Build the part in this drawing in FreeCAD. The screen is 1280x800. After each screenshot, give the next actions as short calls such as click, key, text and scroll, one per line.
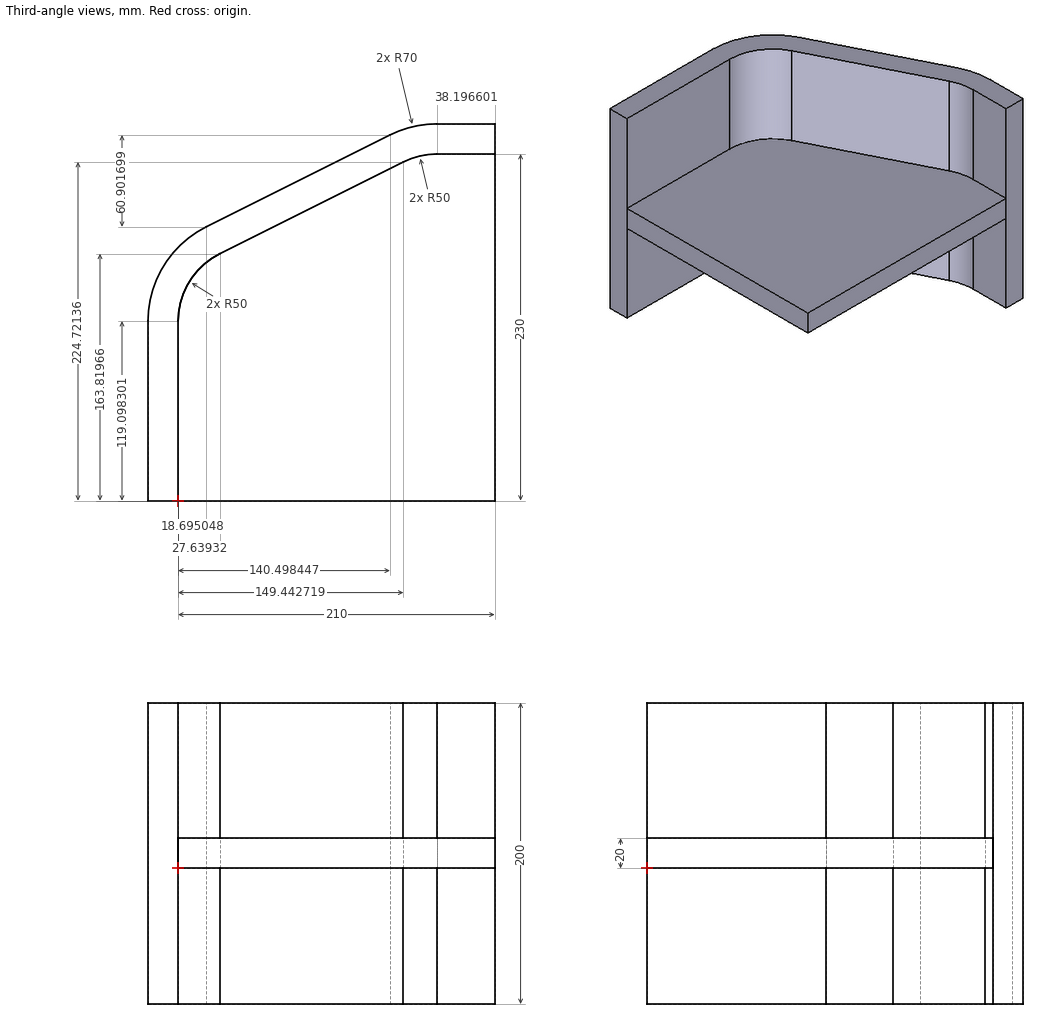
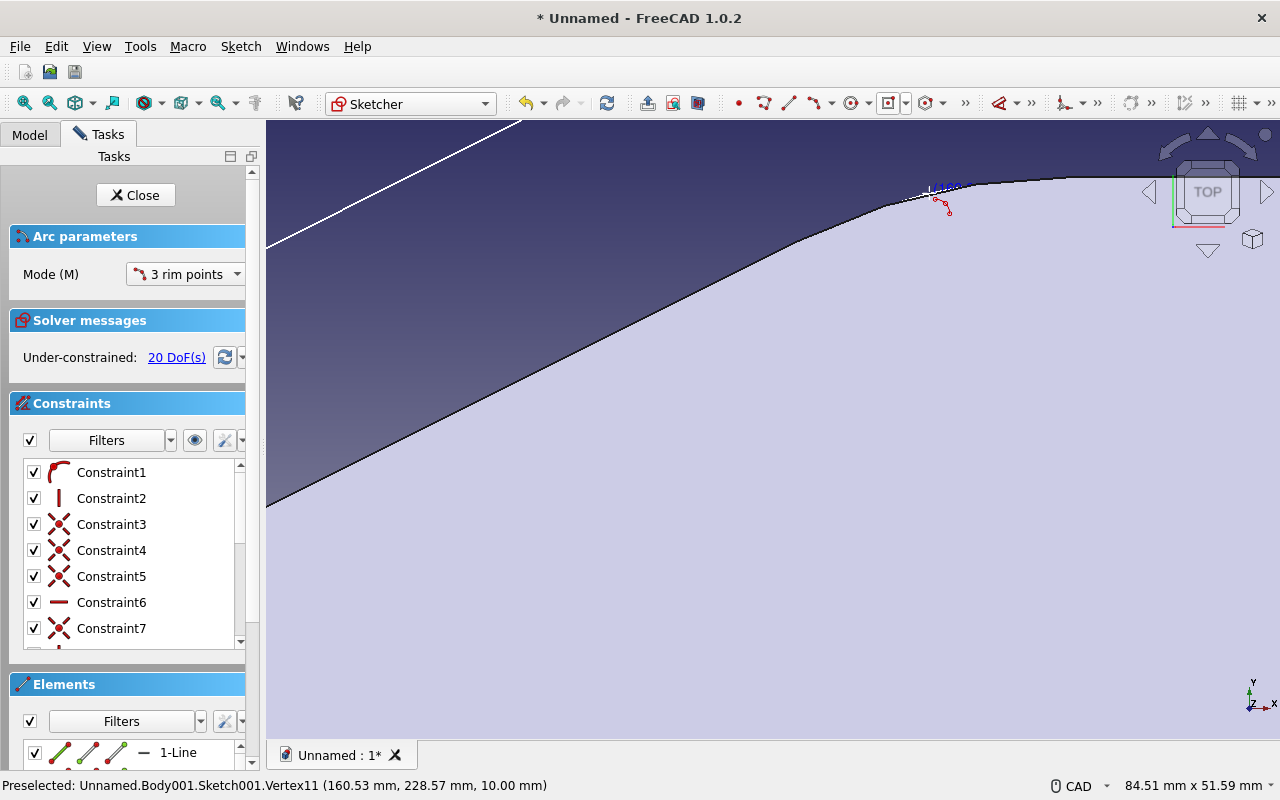
scroll(792, 272, down, 10)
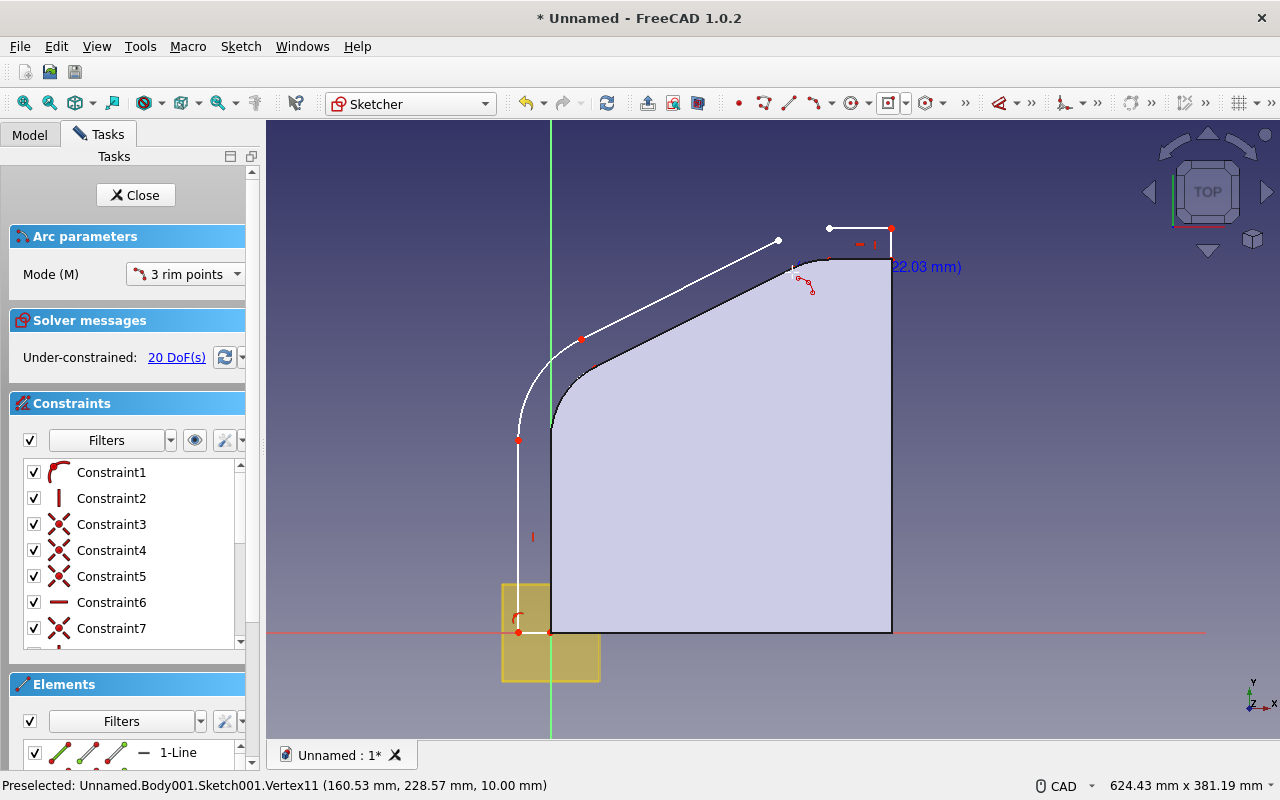
click(829, 228)
click(778, 240)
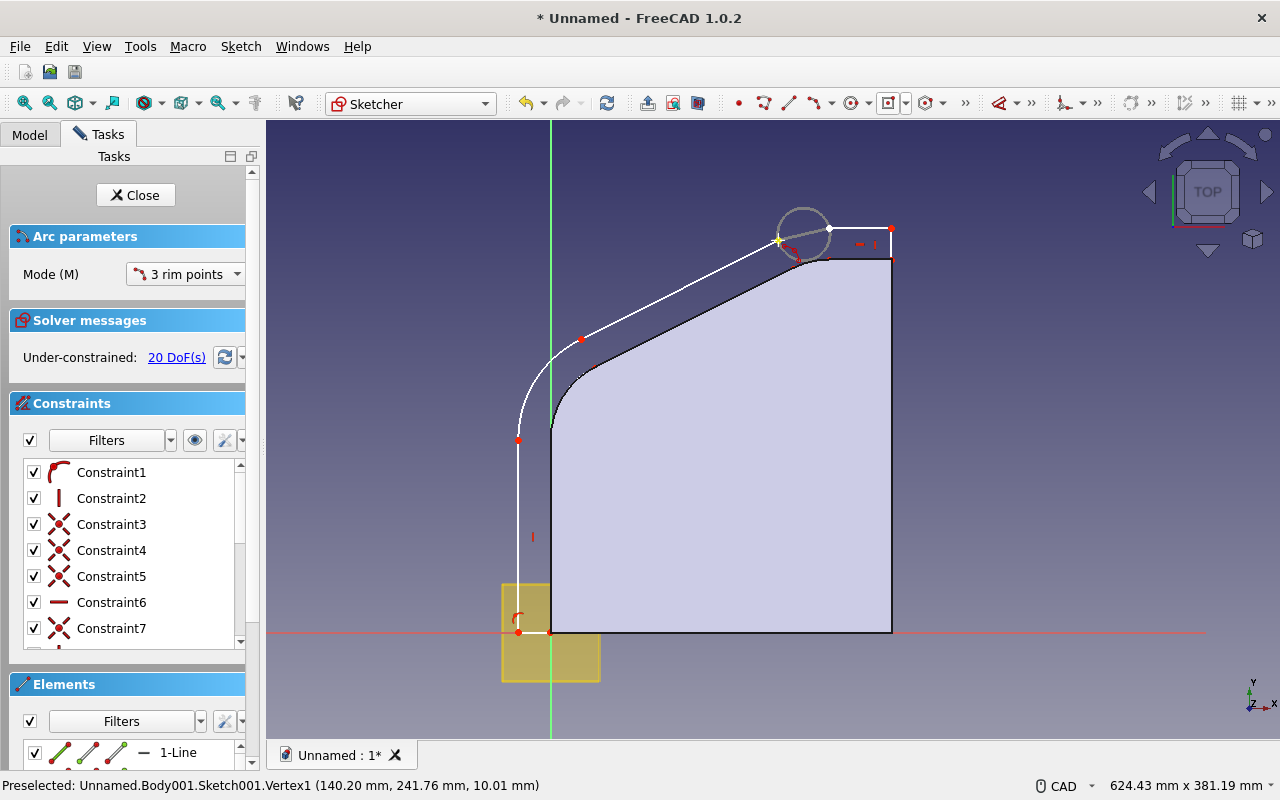
scroll(804, 230, up, 9)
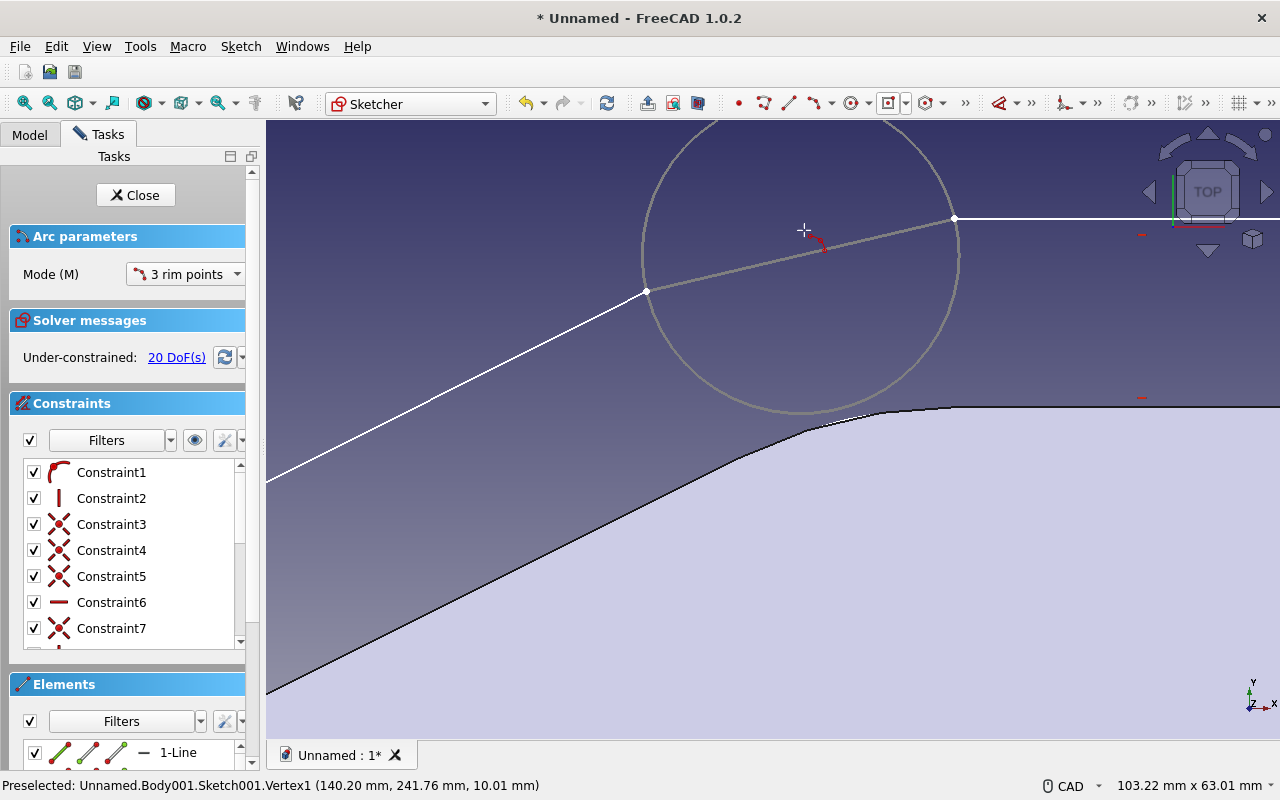
click(799, 229)
key(Escape)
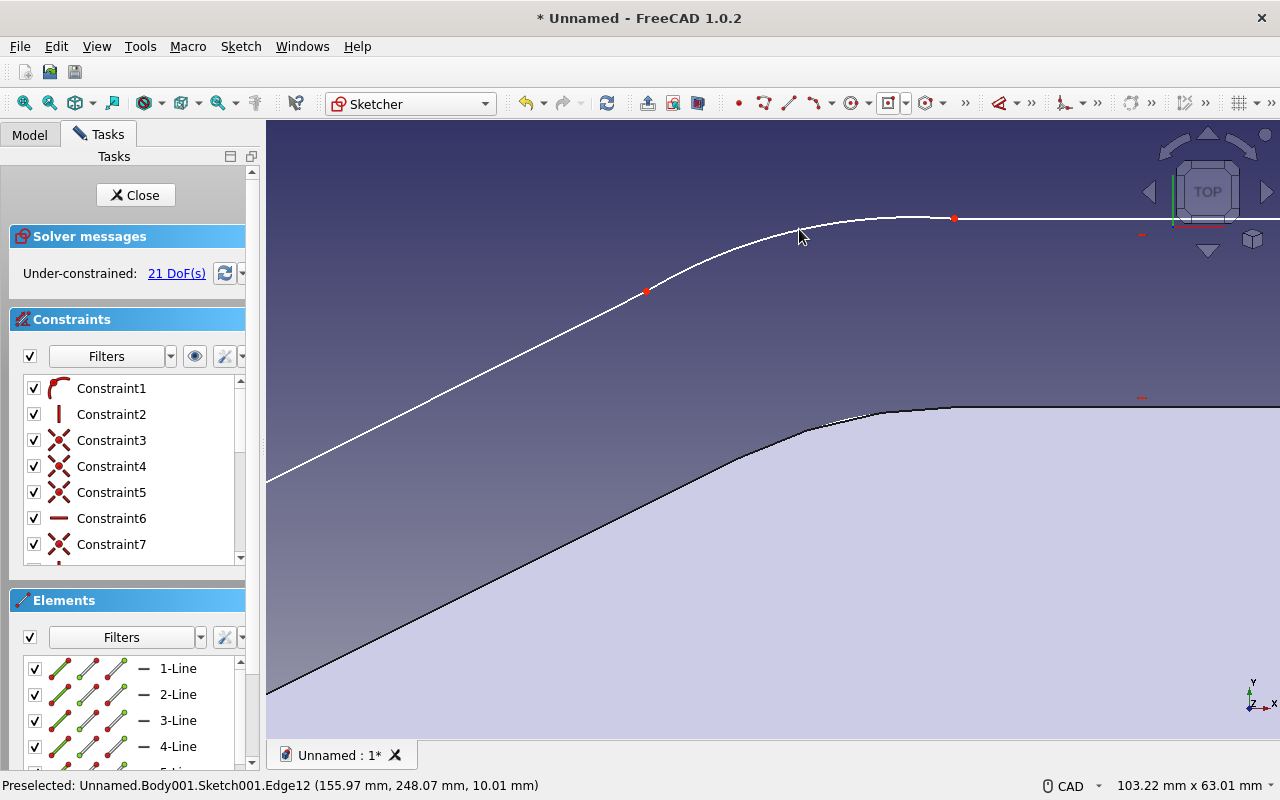
scroll(804, 230, down, 9)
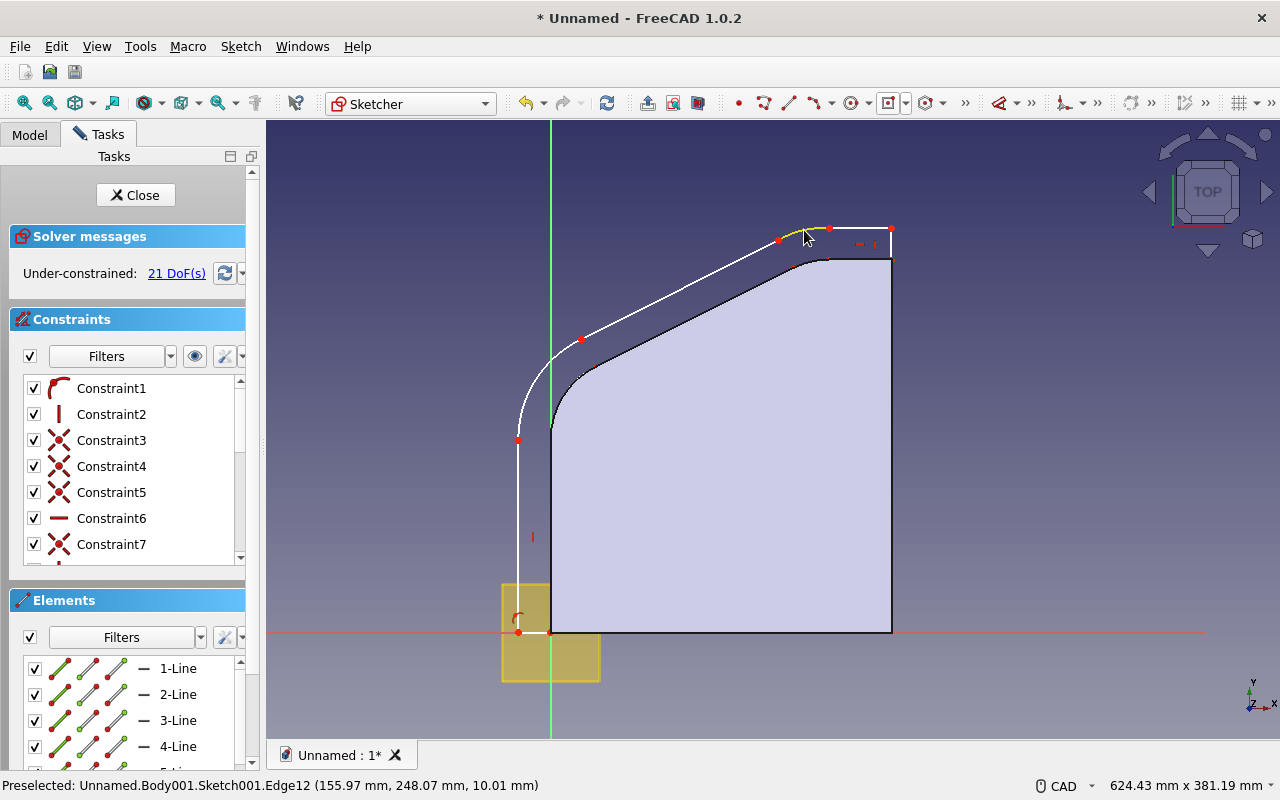
scroll(553, 575, up, 9)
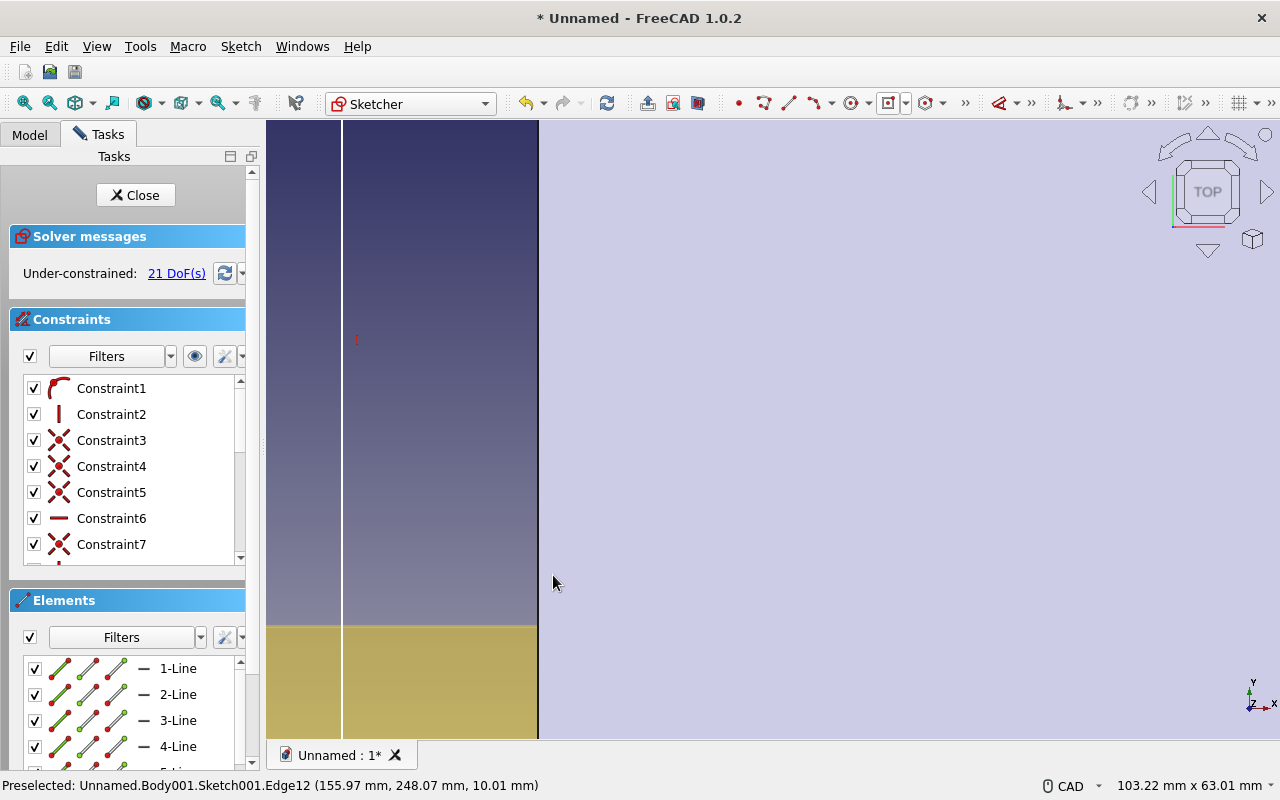
click(554, 572)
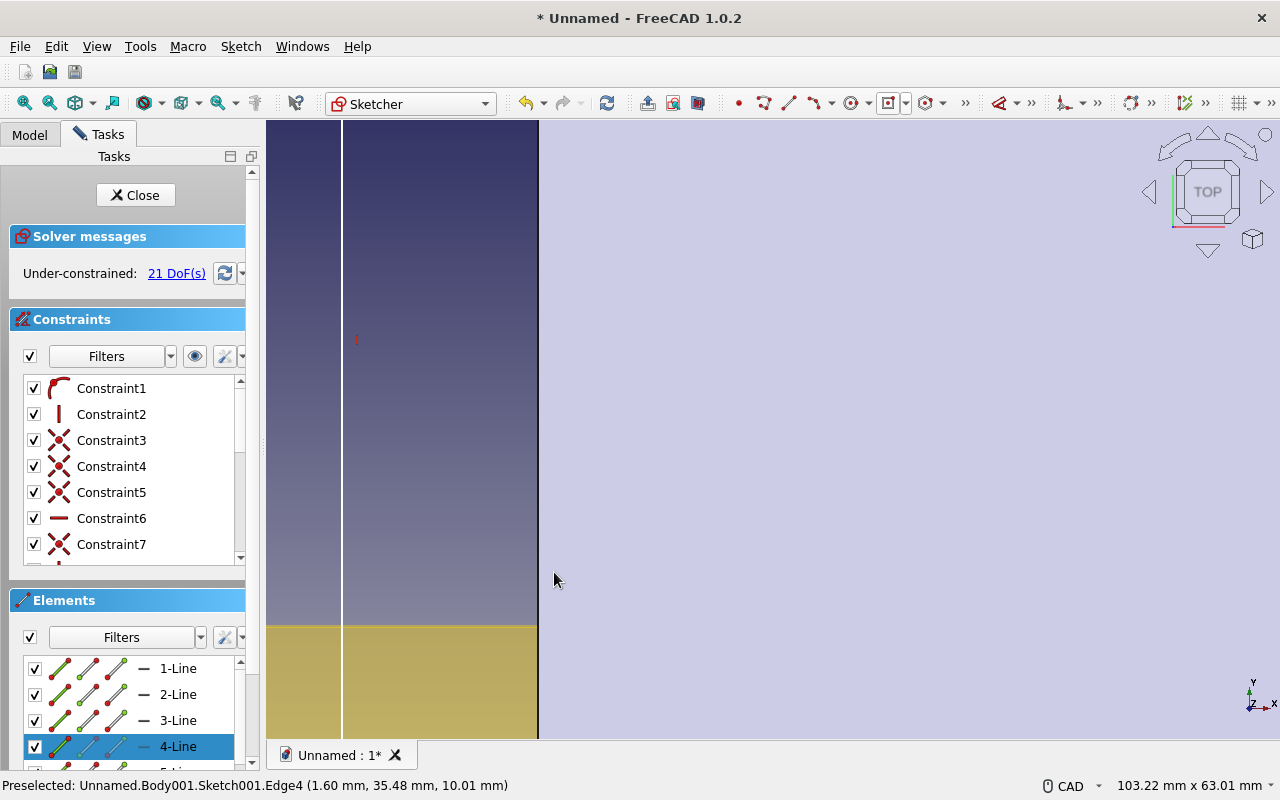
key(v)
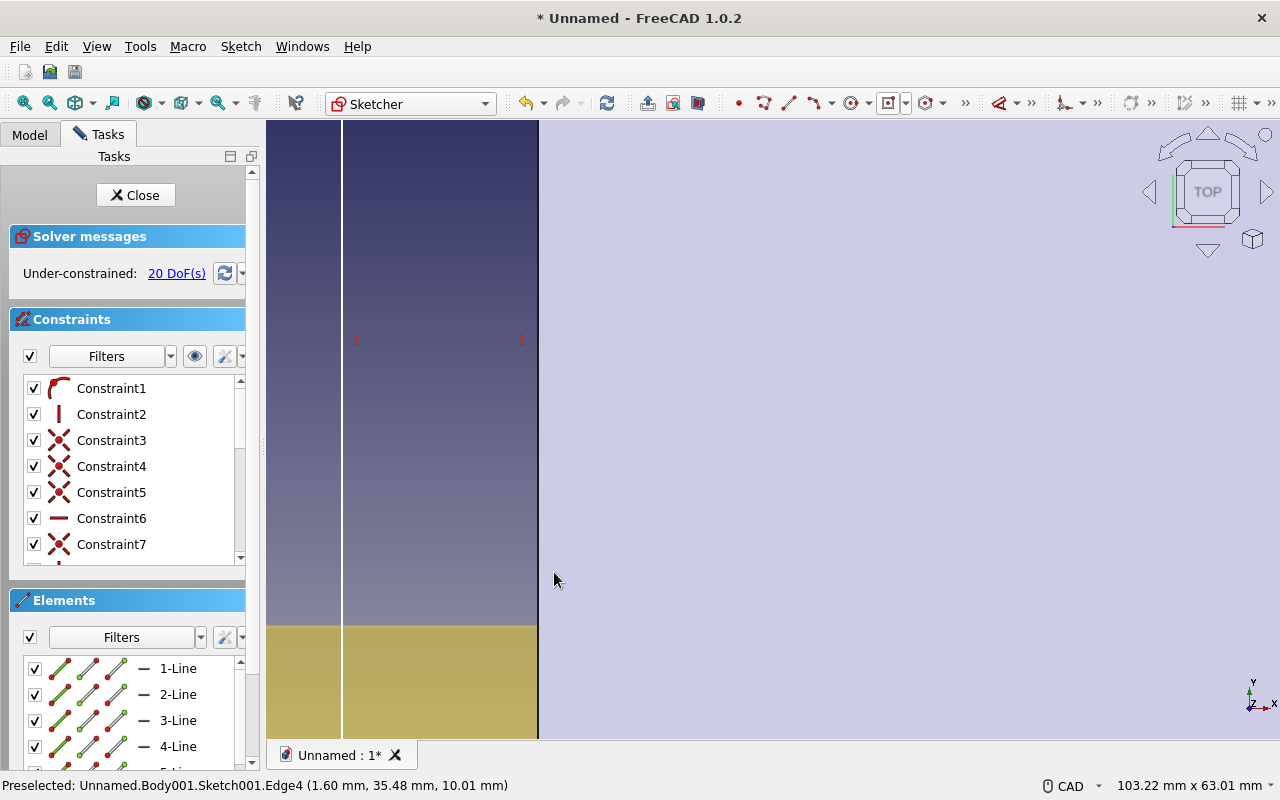
scroll(553, 575, down, 9)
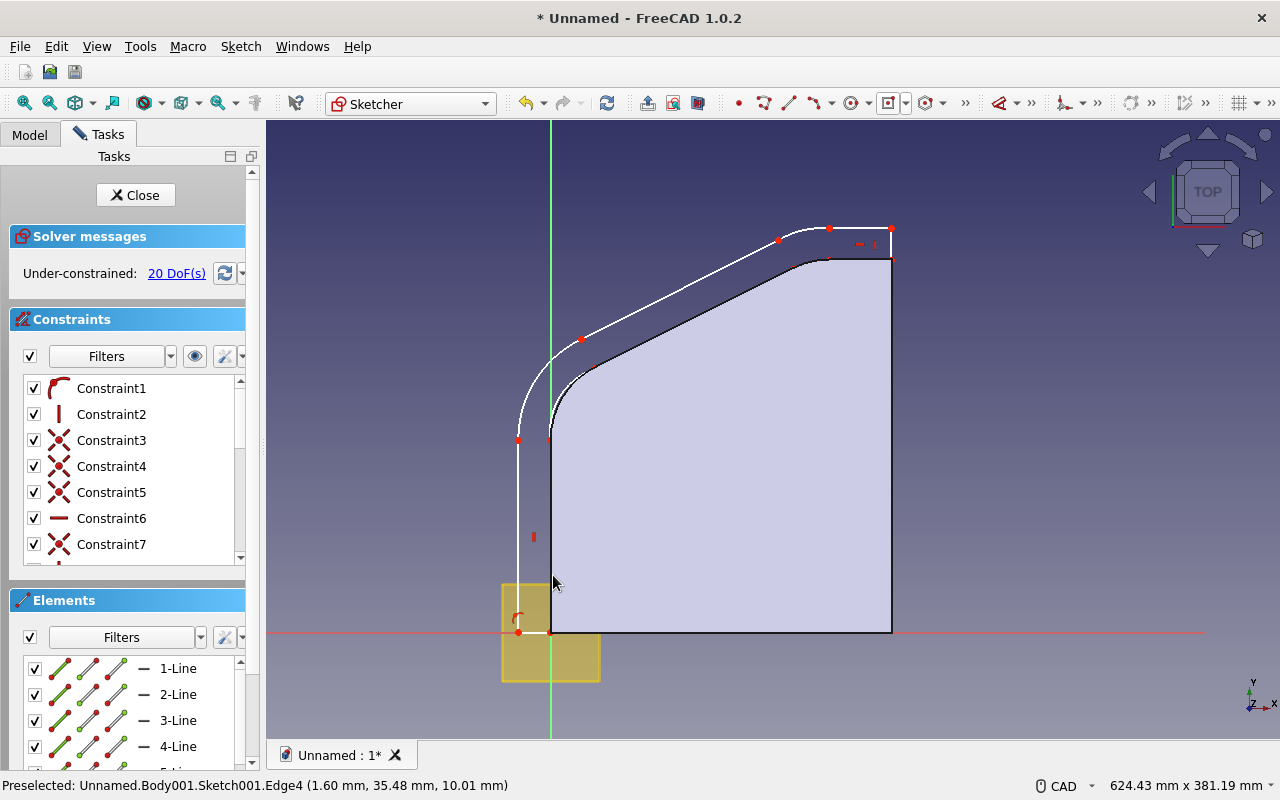
click(551, 361)